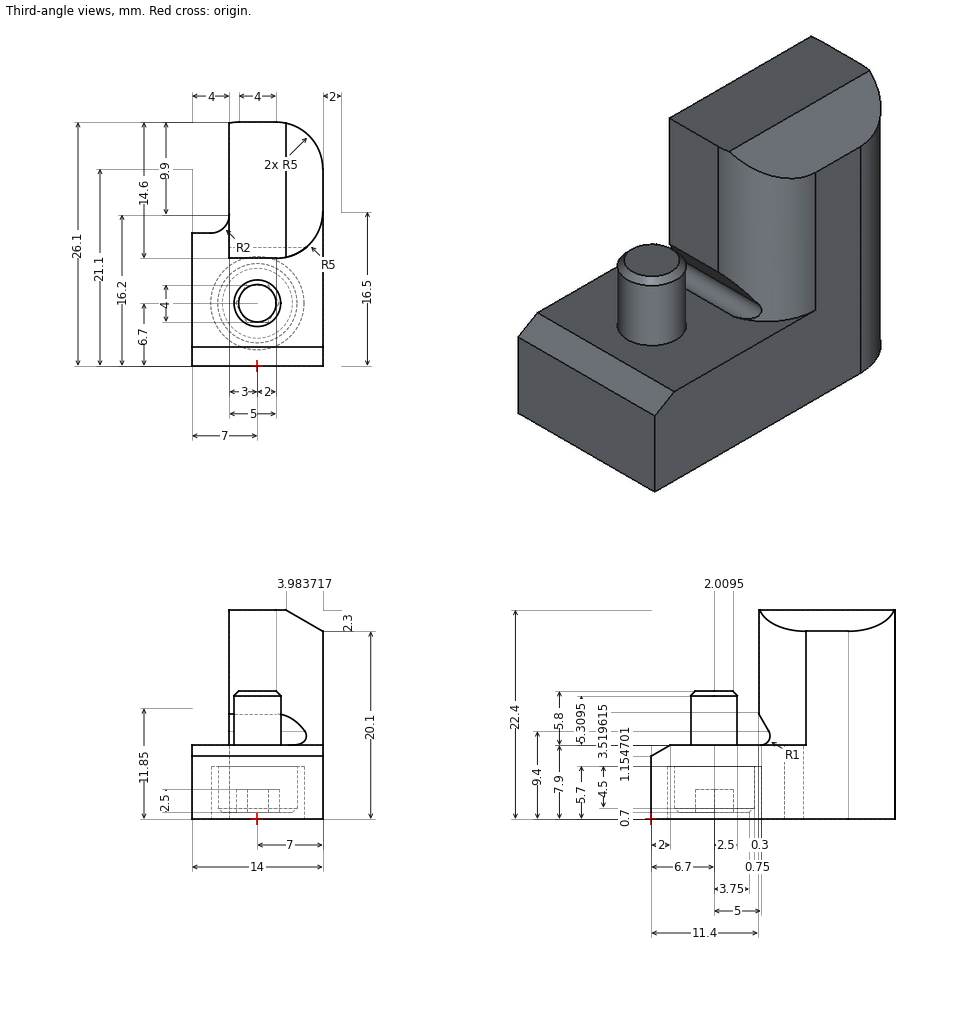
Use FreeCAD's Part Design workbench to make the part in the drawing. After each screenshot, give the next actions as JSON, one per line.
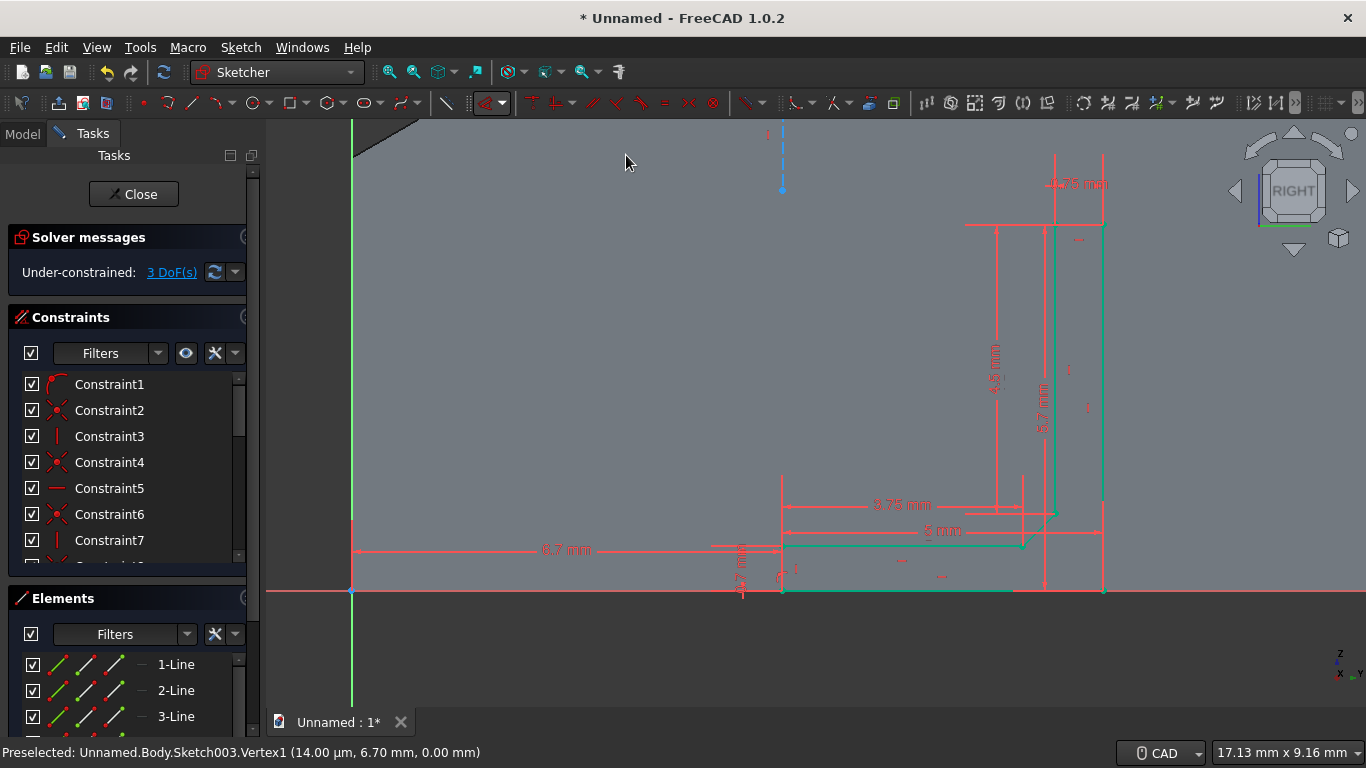
{"action": "left_click", "coordinate": [783, 190]}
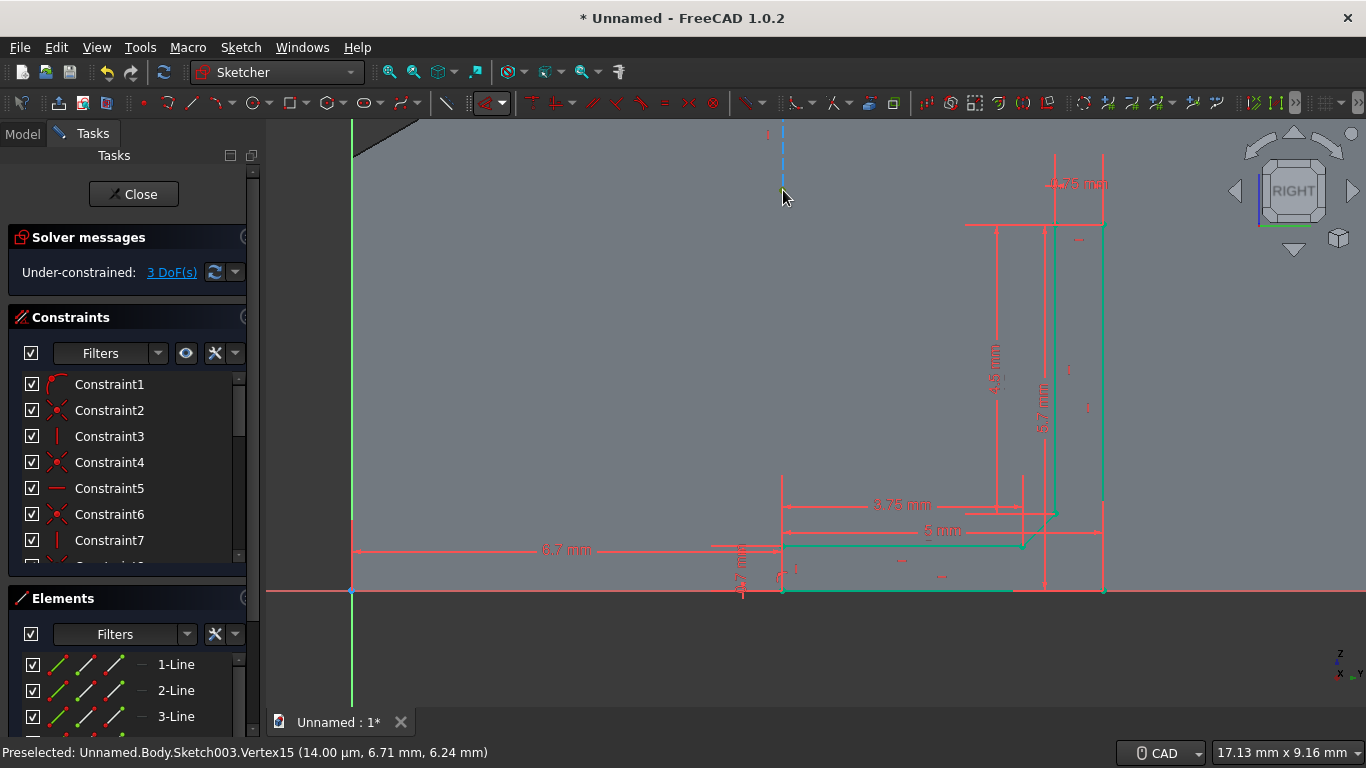
{"action": "left_click", "coordinate": [504, 104]}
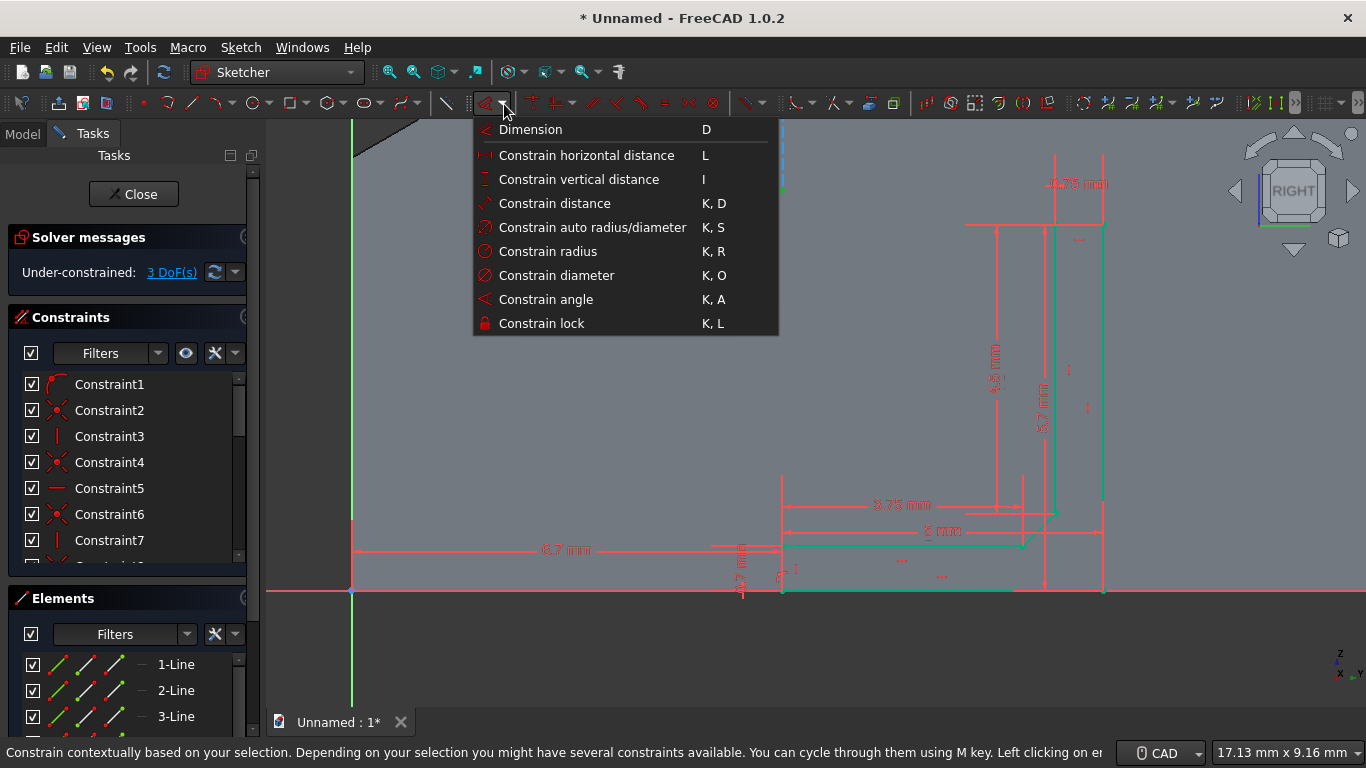
{"action": "left_click", "coordinate": [626, 155]}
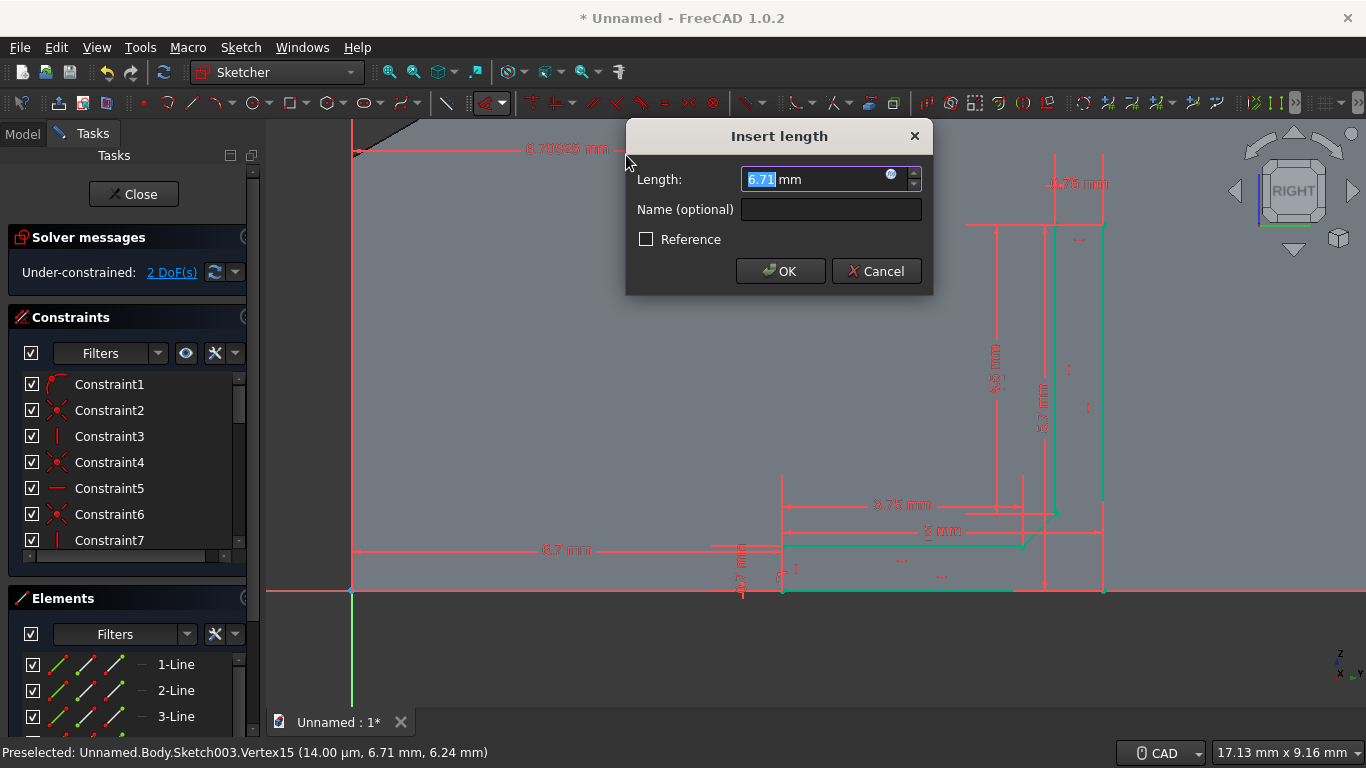
{"action": "type", "text": "6.7"}
{"action": "key", "text": "Return"}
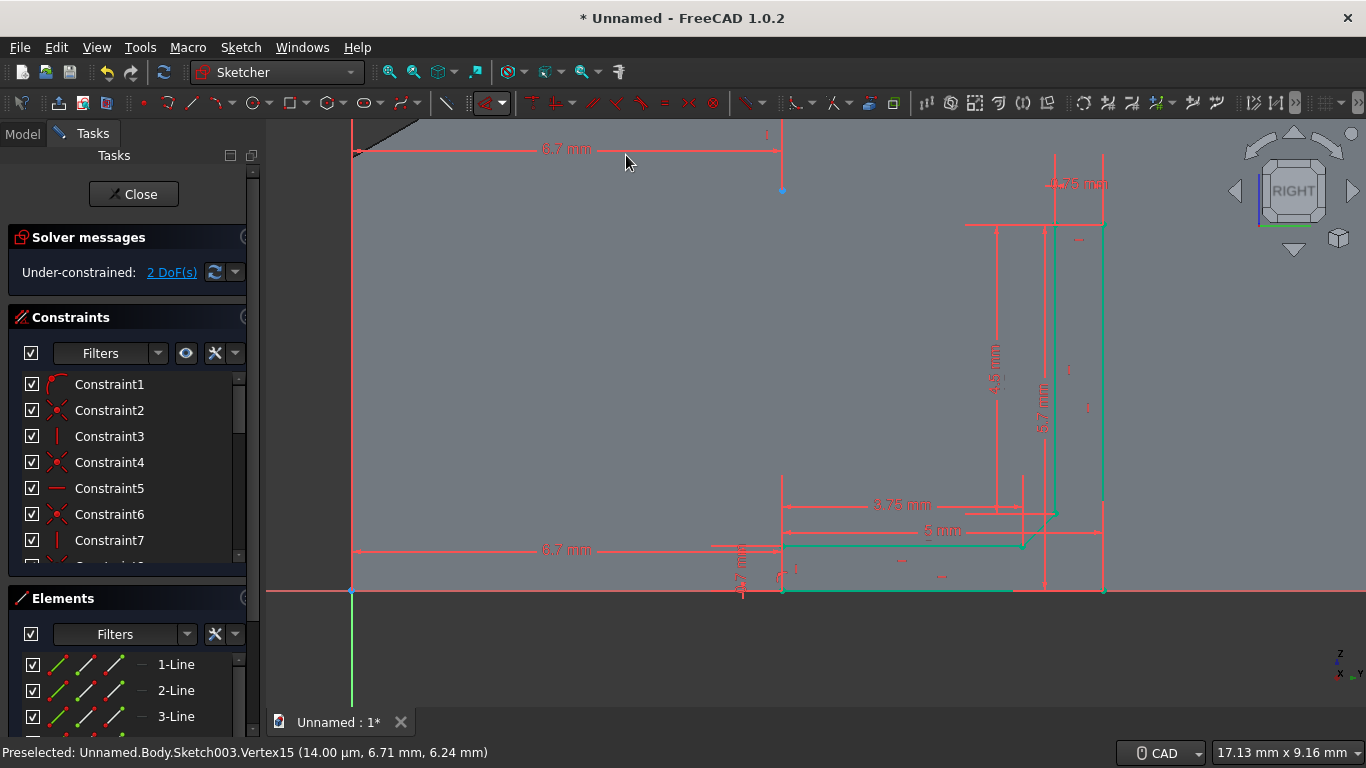
{"action": "left_click", "coordinate": [134, 194]}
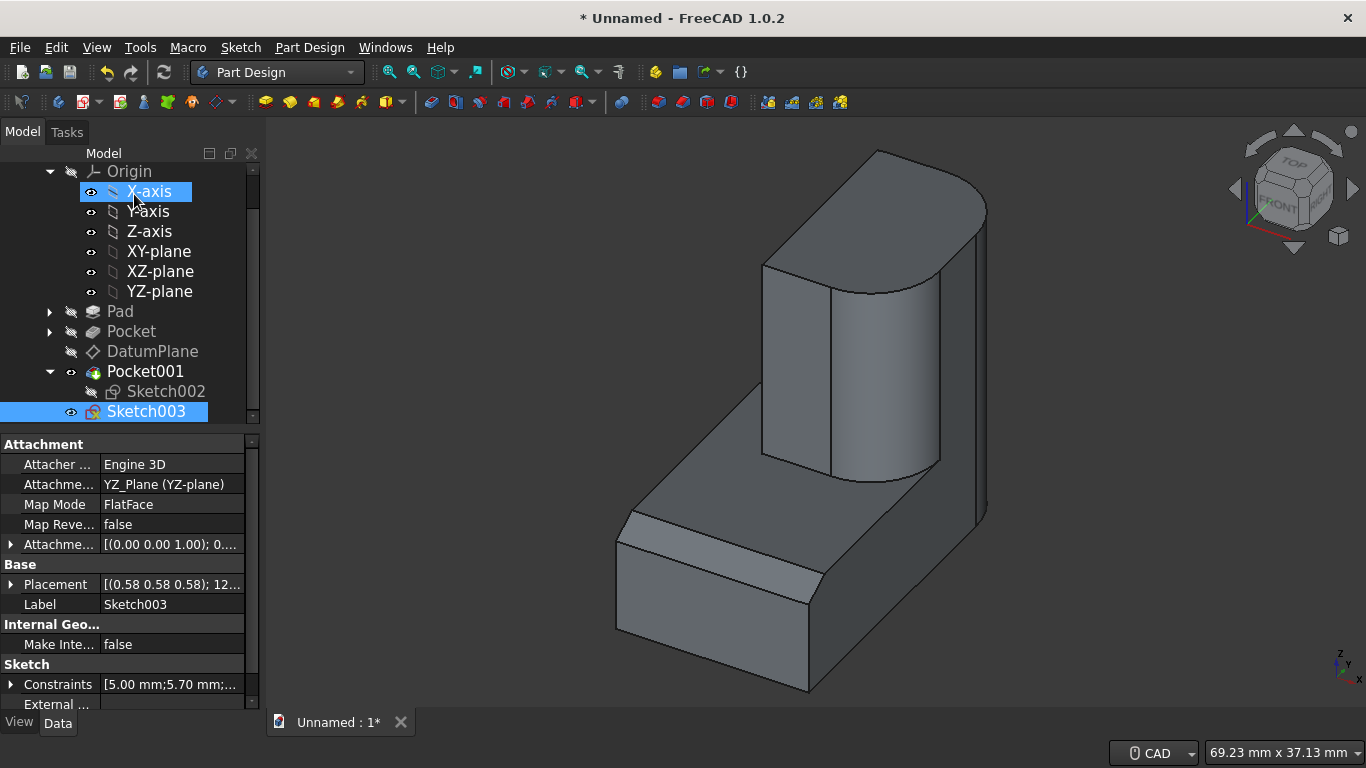
{"action": "left_click", "coordinate": [480, 102]}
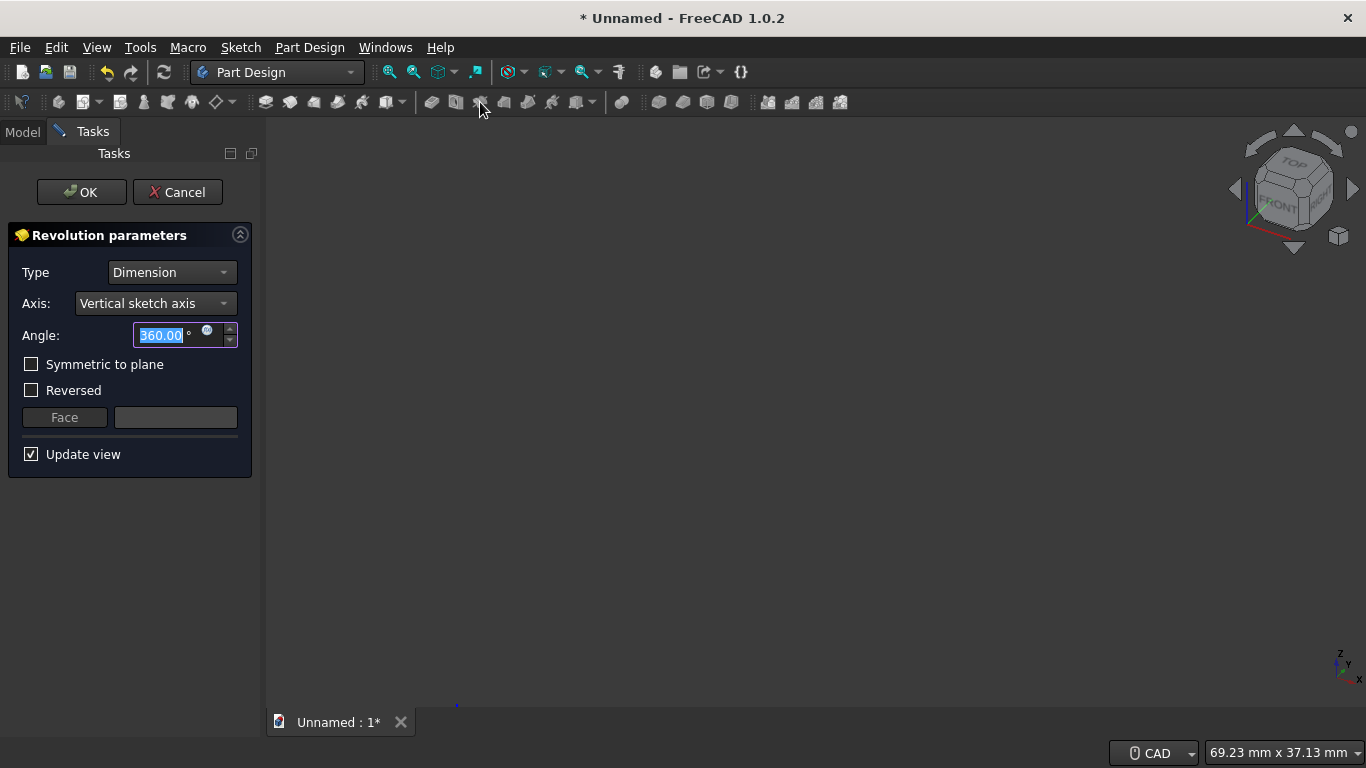
{"action": "left_click", "coordinate": [156, 304]}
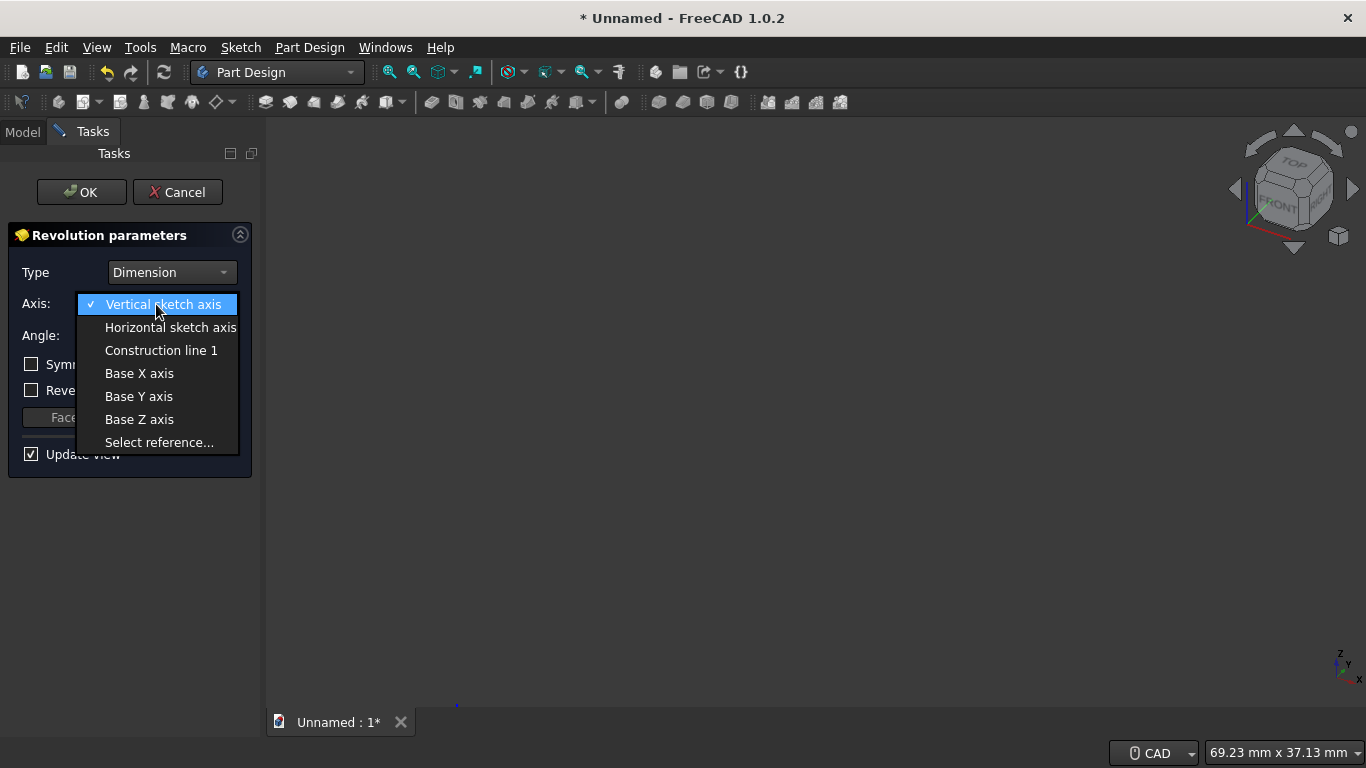
{"action": "left_click", "coordinate": [156, 350]}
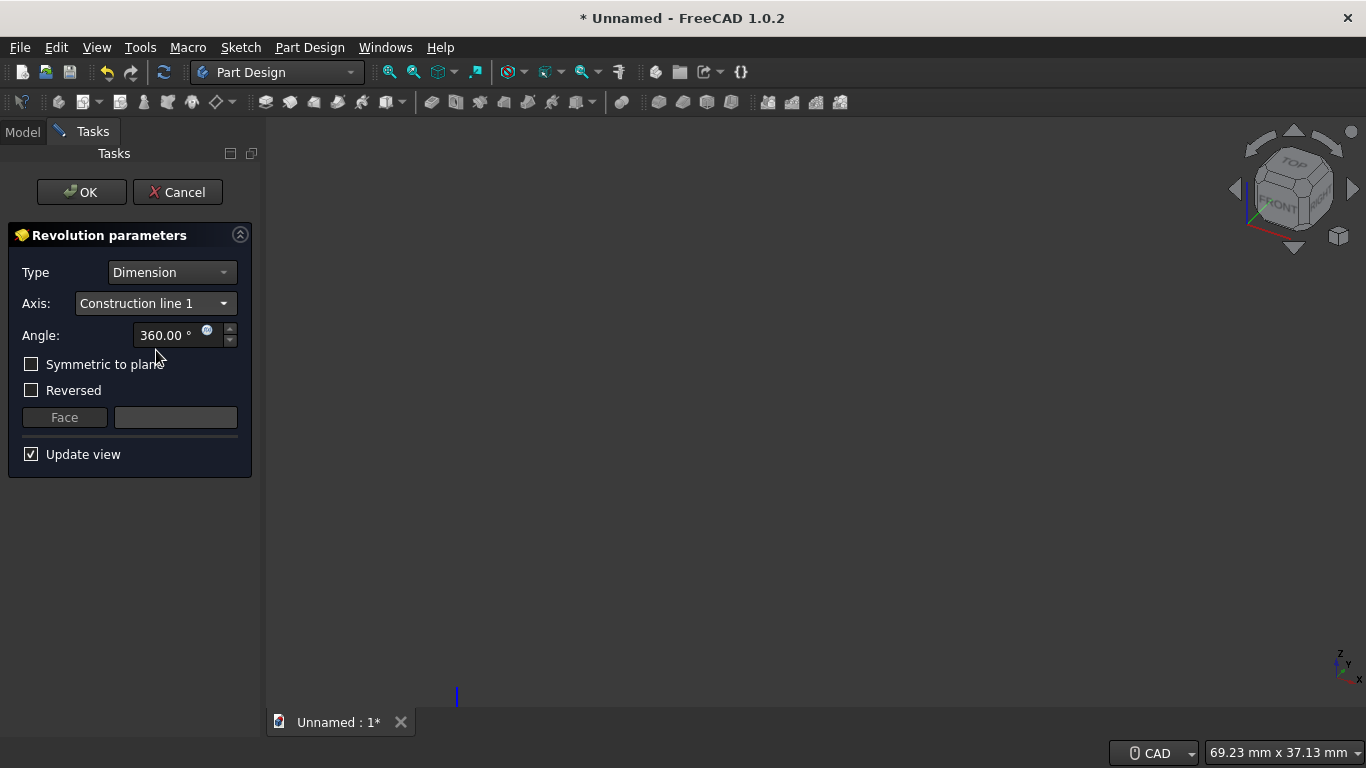
{"action": "left_click", "coordinate": [82, 192]}